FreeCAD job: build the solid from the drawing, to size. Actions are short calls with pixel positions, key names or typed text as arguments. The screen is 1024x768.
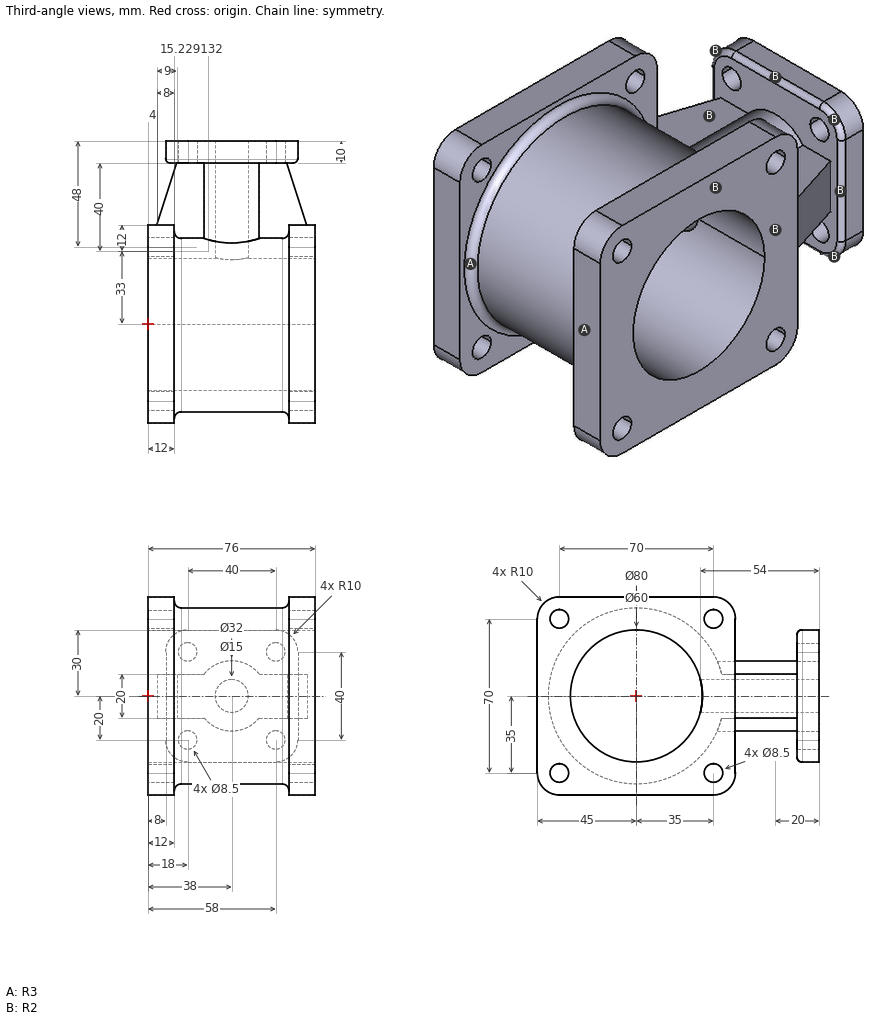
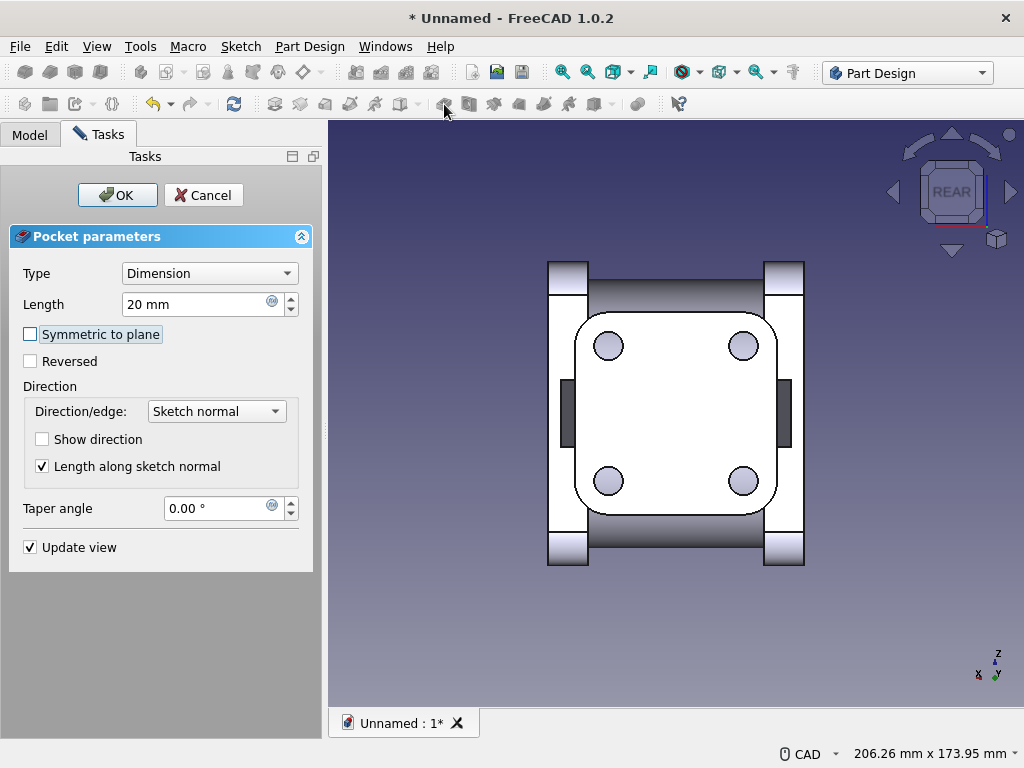
click(118, 195)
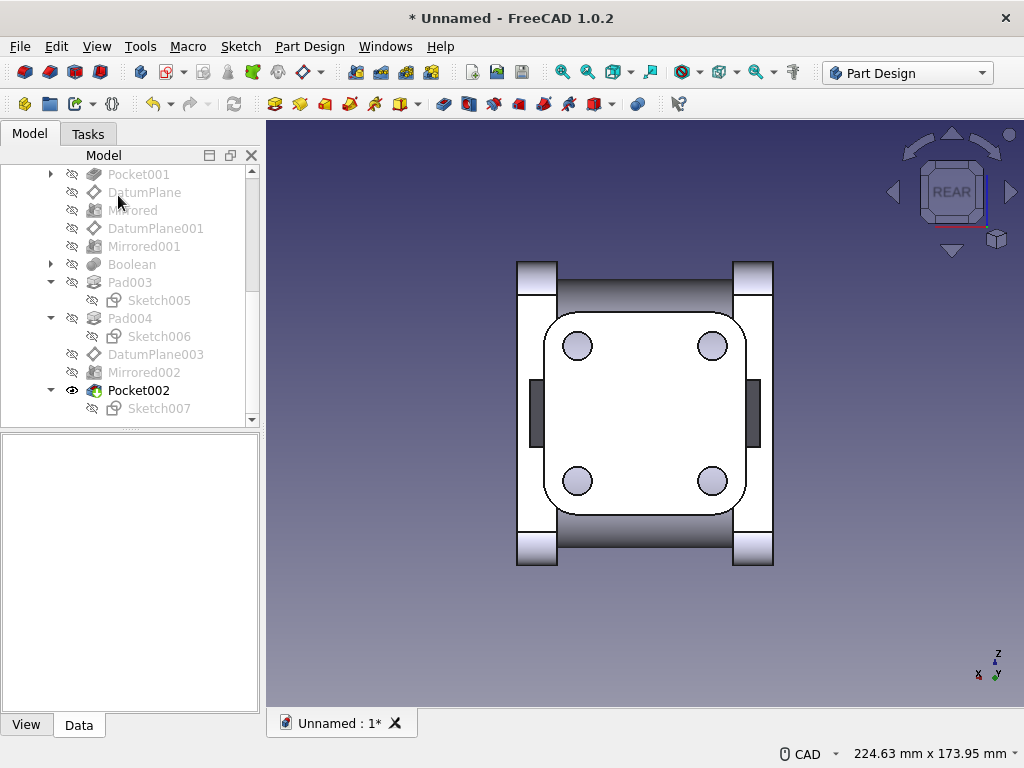
click(645, 412)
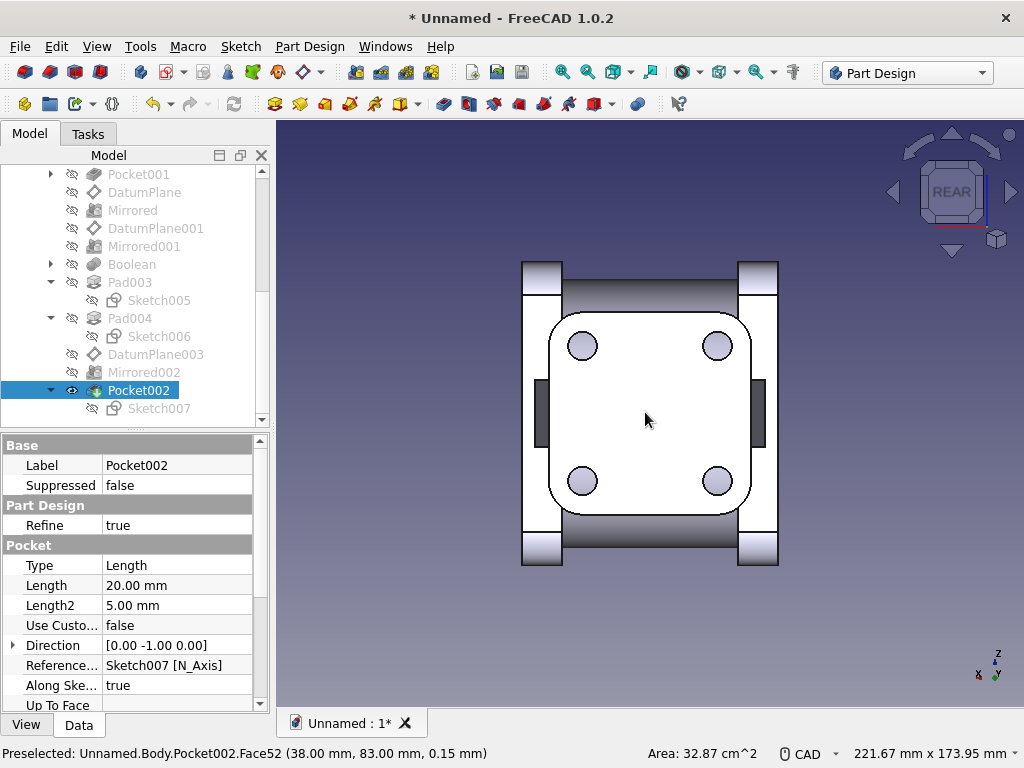
click(166, 72)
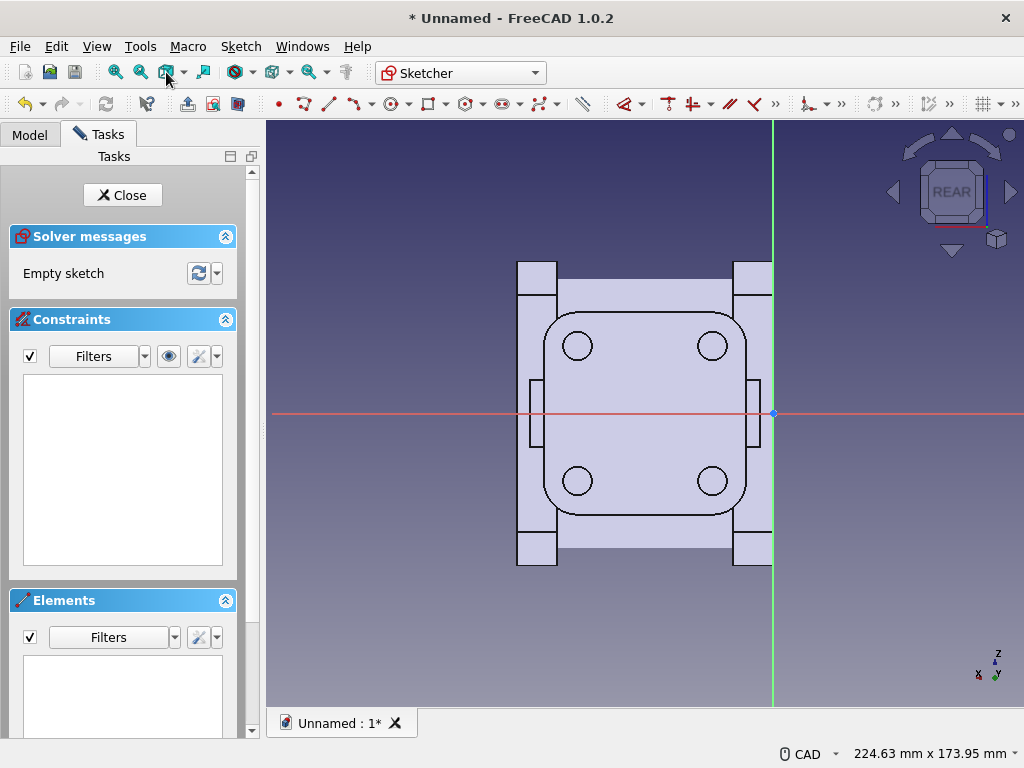
scroll(656, 414, up, 10)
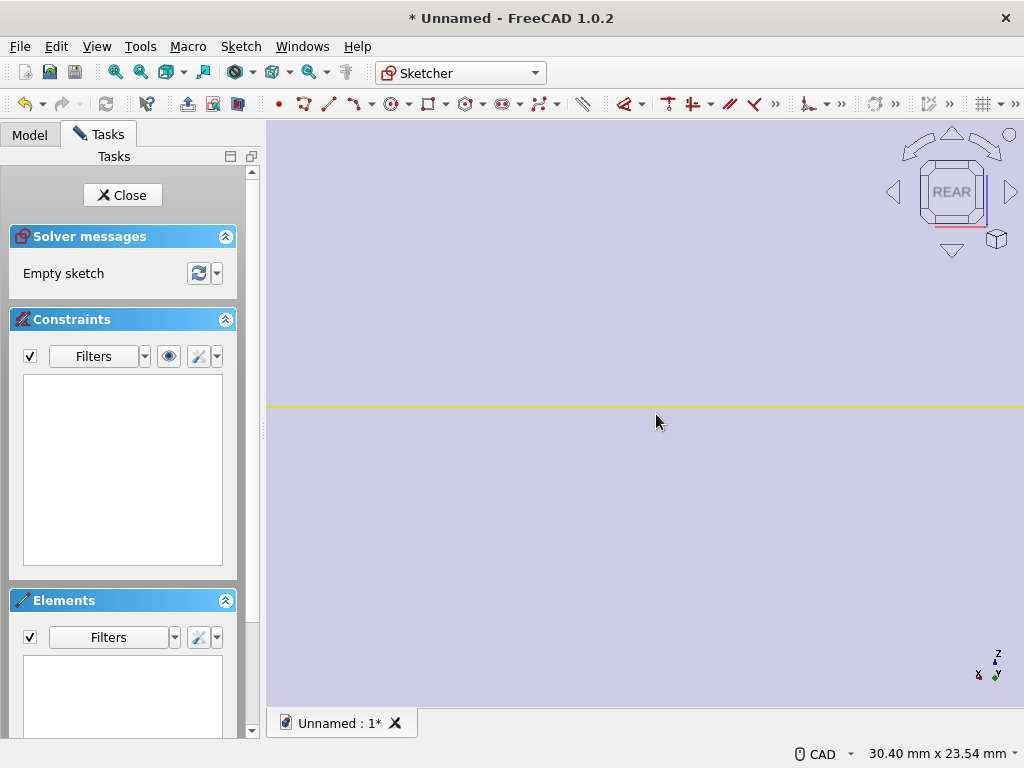
key(g)
key(c)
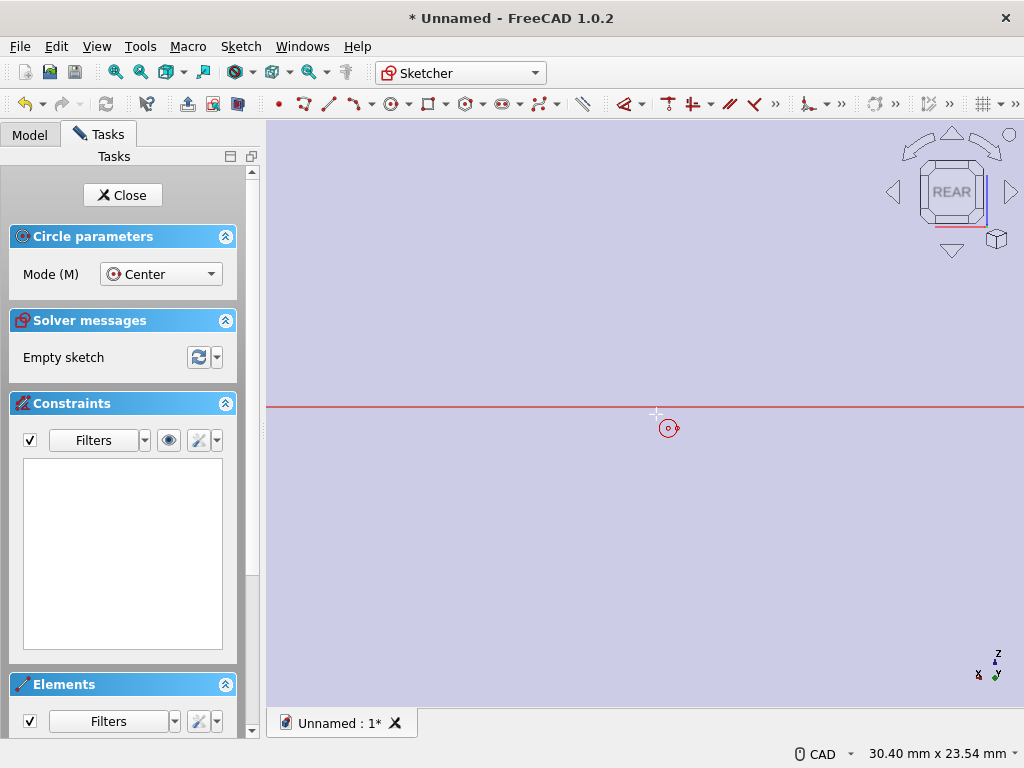
click(571, 407)
click(704, 275)
key(Escape)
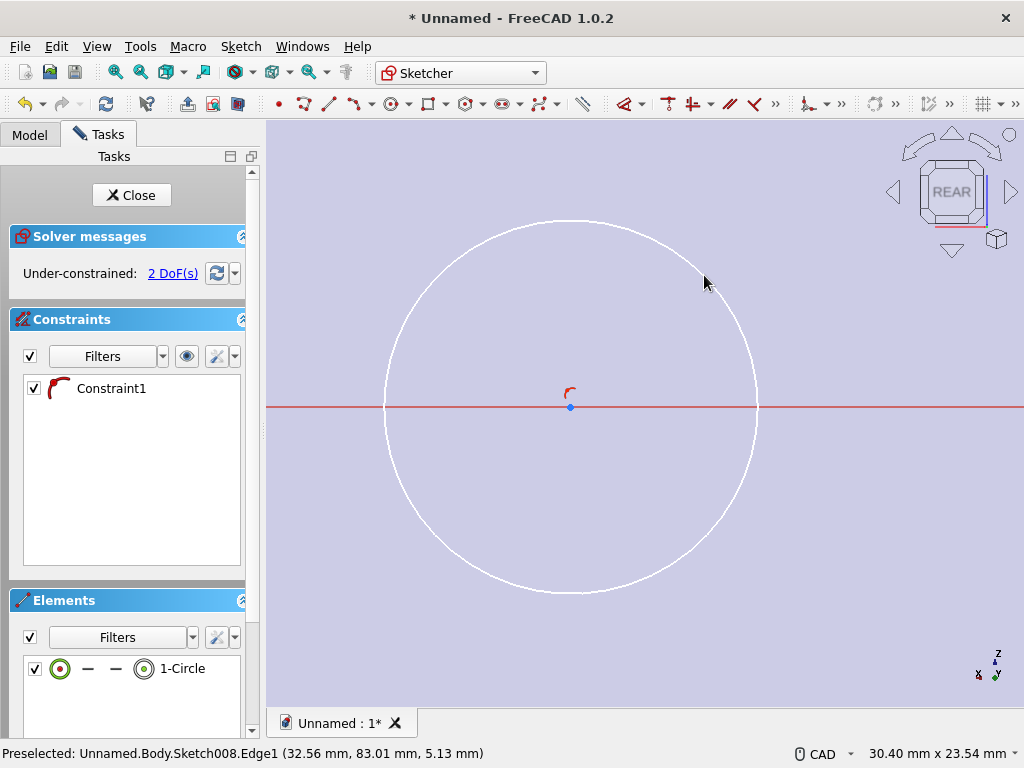
click(624, 104)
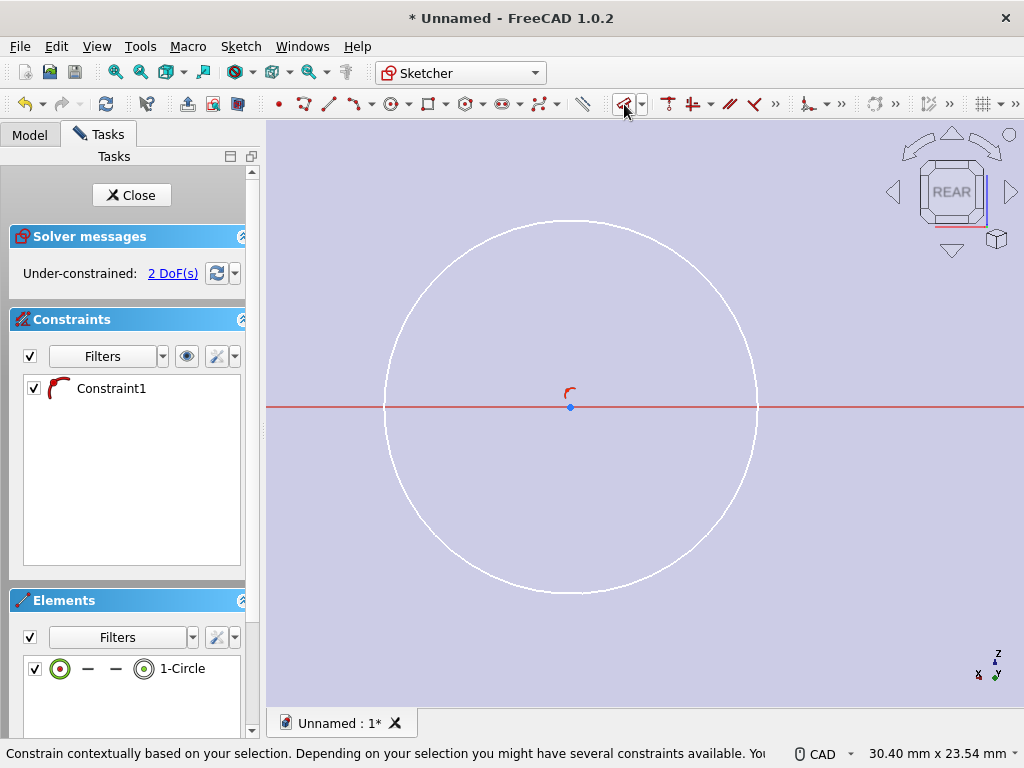
click(703, 275)
click(726, 252)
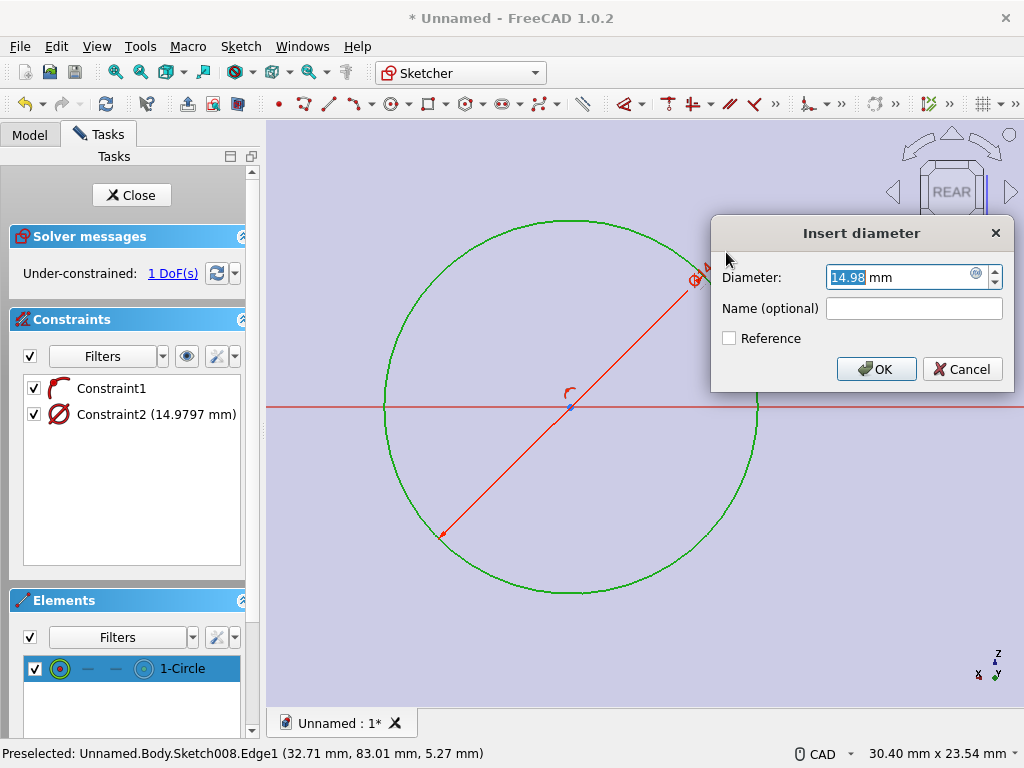
text(15)
key(Return)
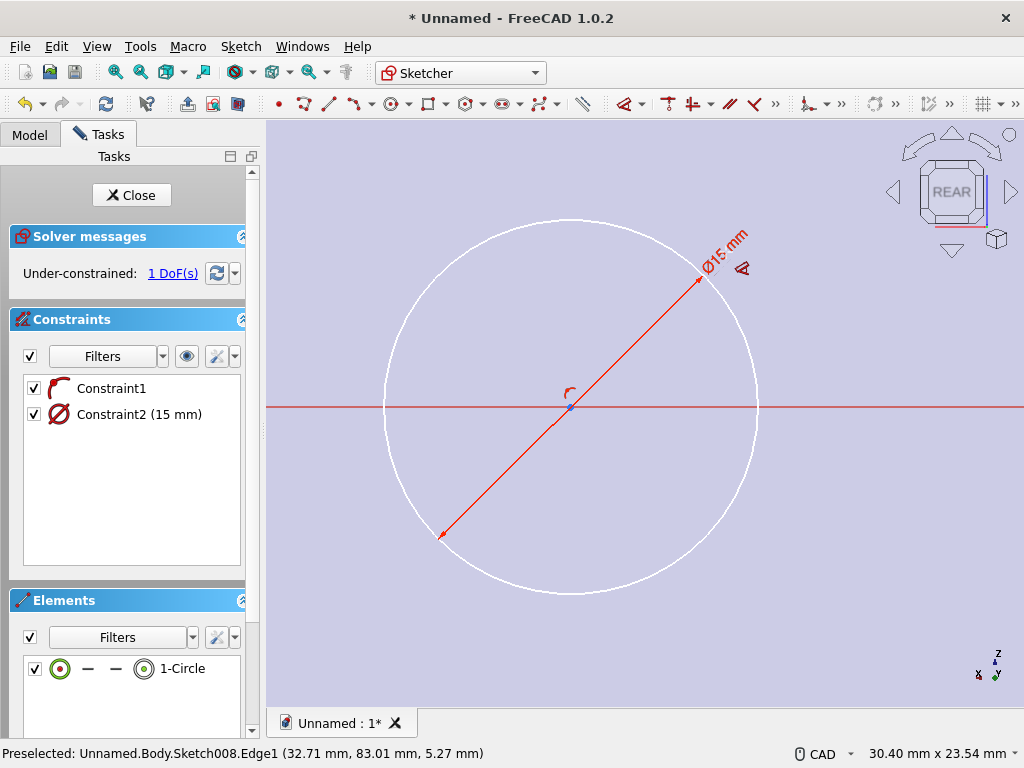
click(571, 407)
click(715, 441)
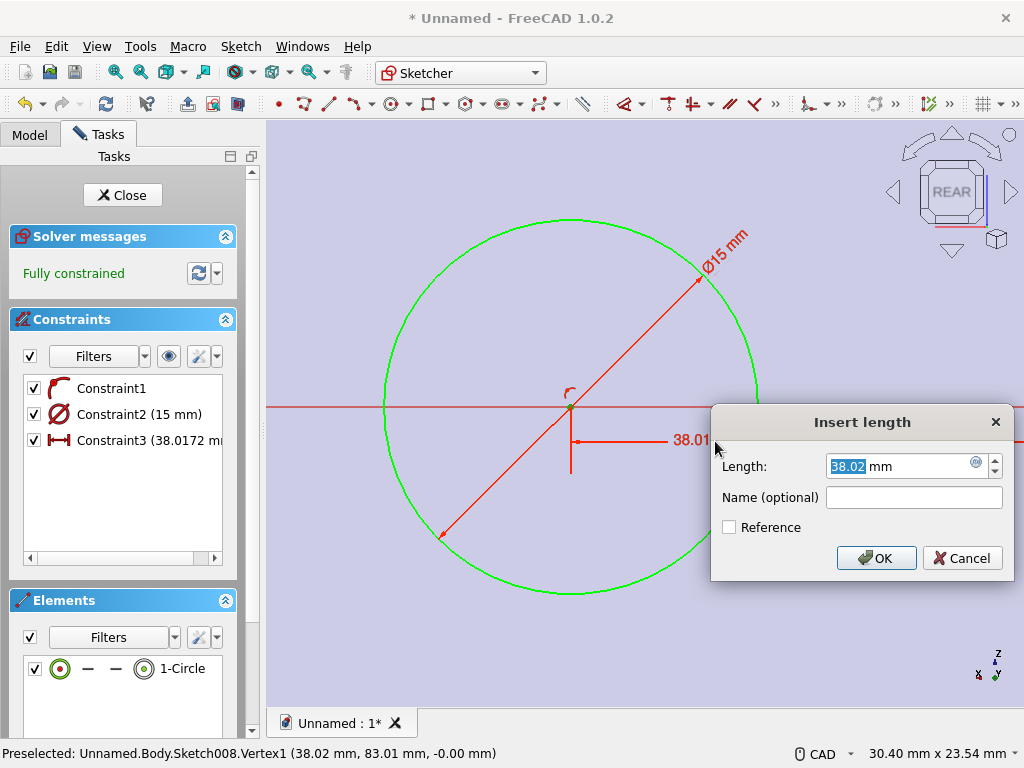
text(38)
key(Return)
key(Escape)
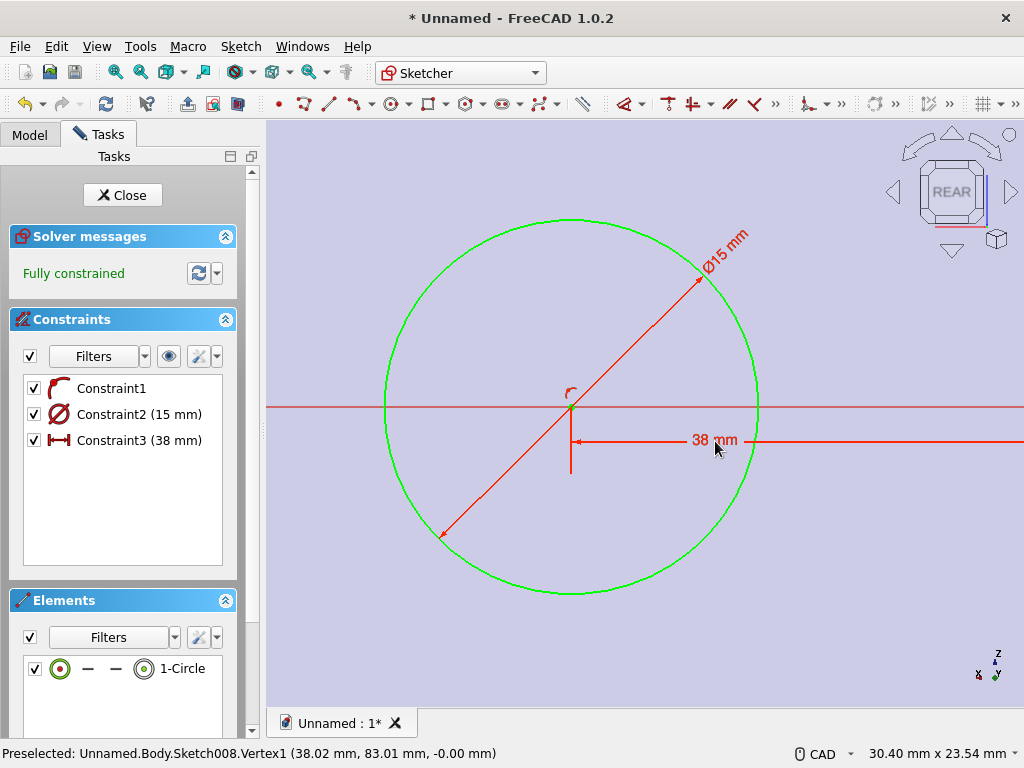
click(123, 195)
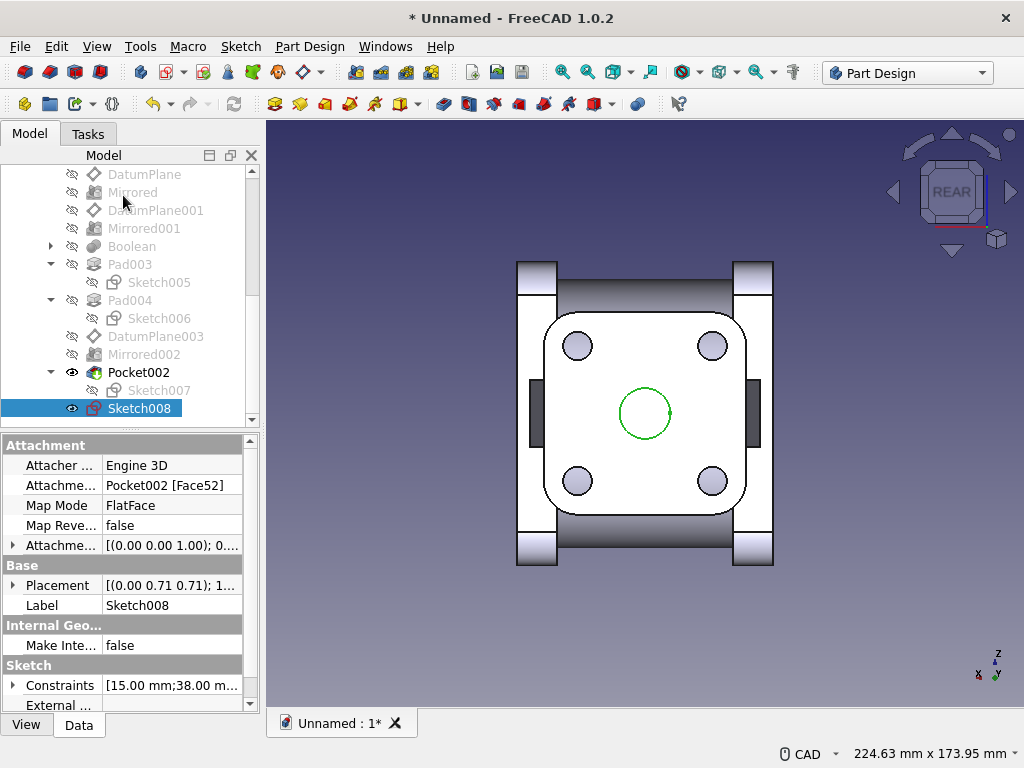
click(444, 104)